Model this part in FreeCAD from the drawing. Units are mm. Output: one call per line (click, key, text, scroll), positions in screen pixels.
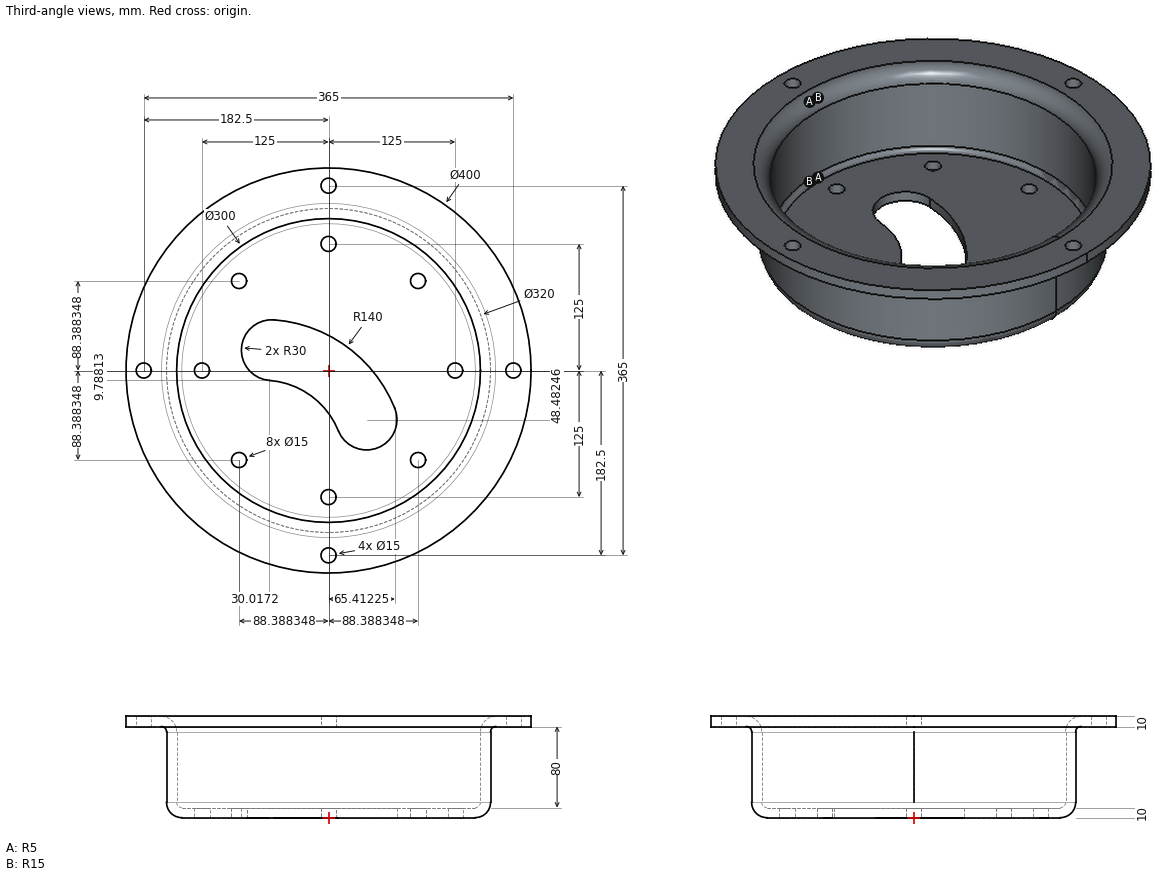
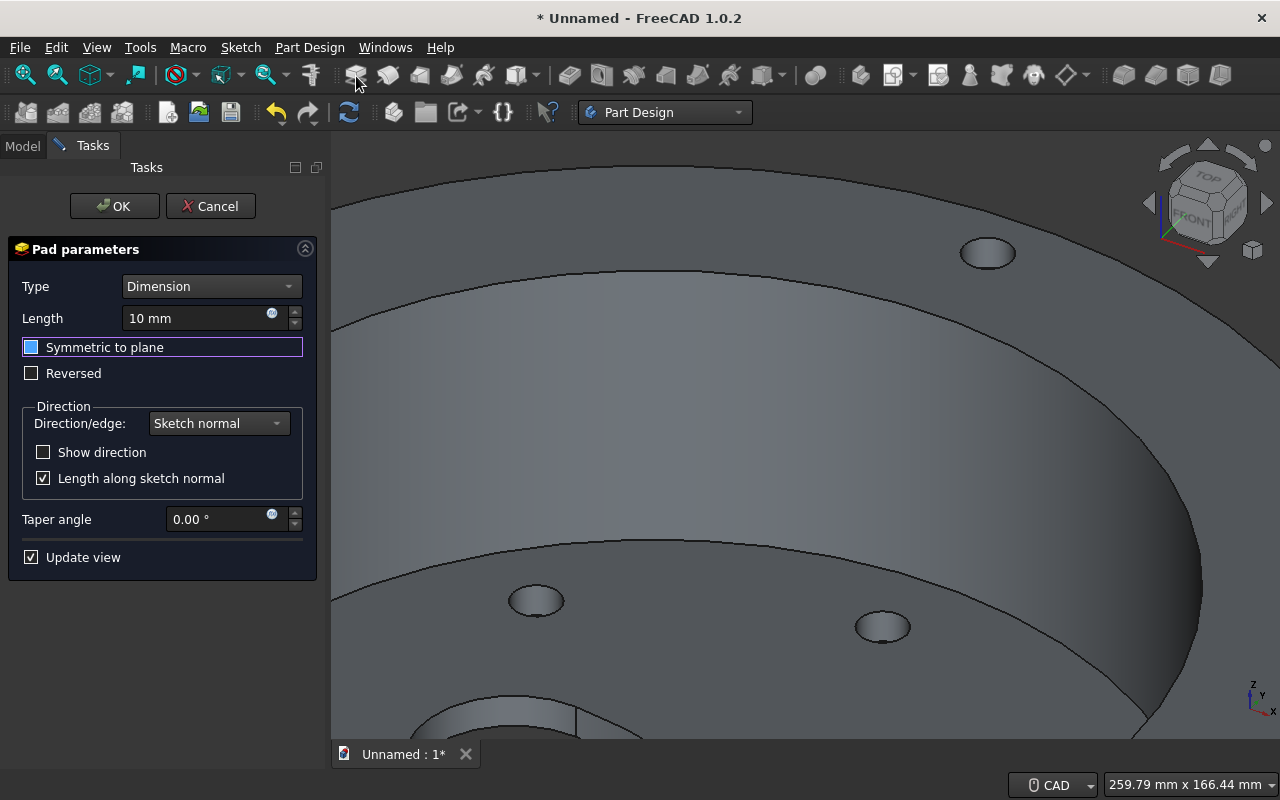
click(115, 206)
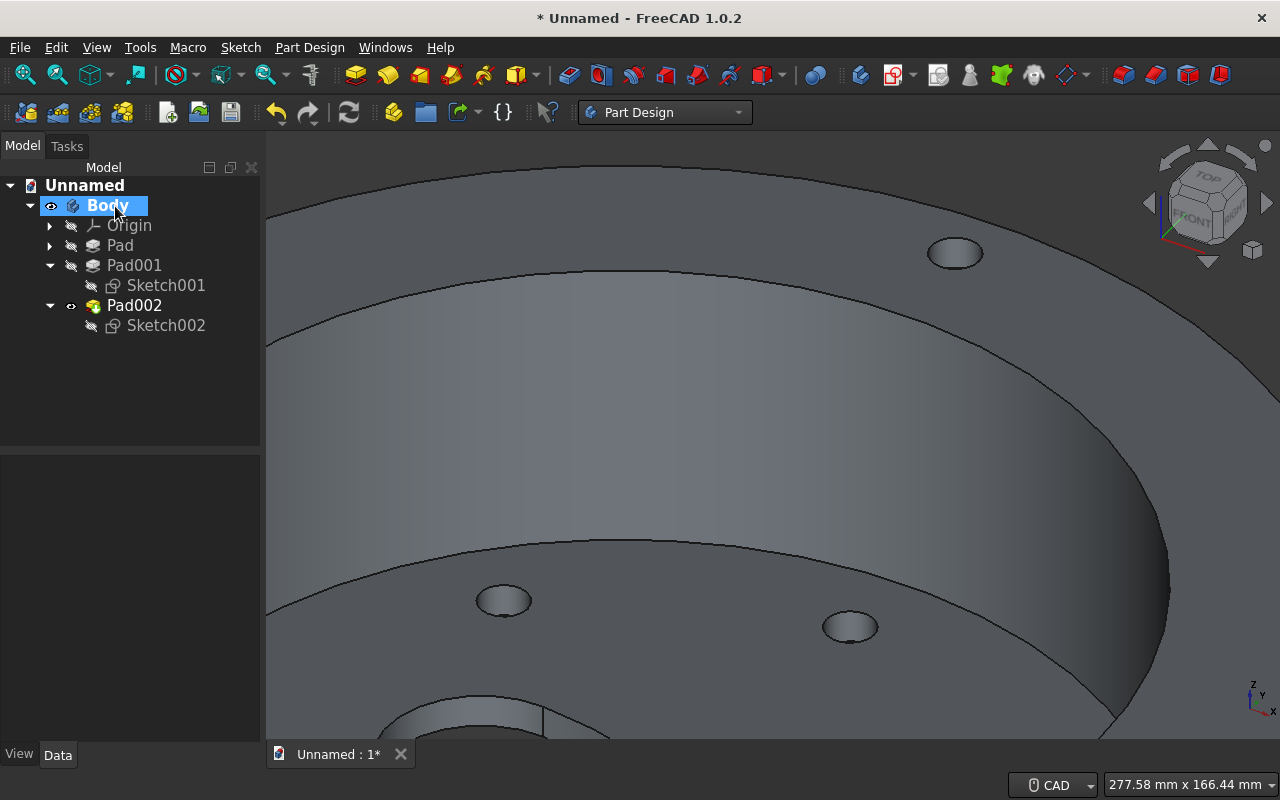
click(26, 76)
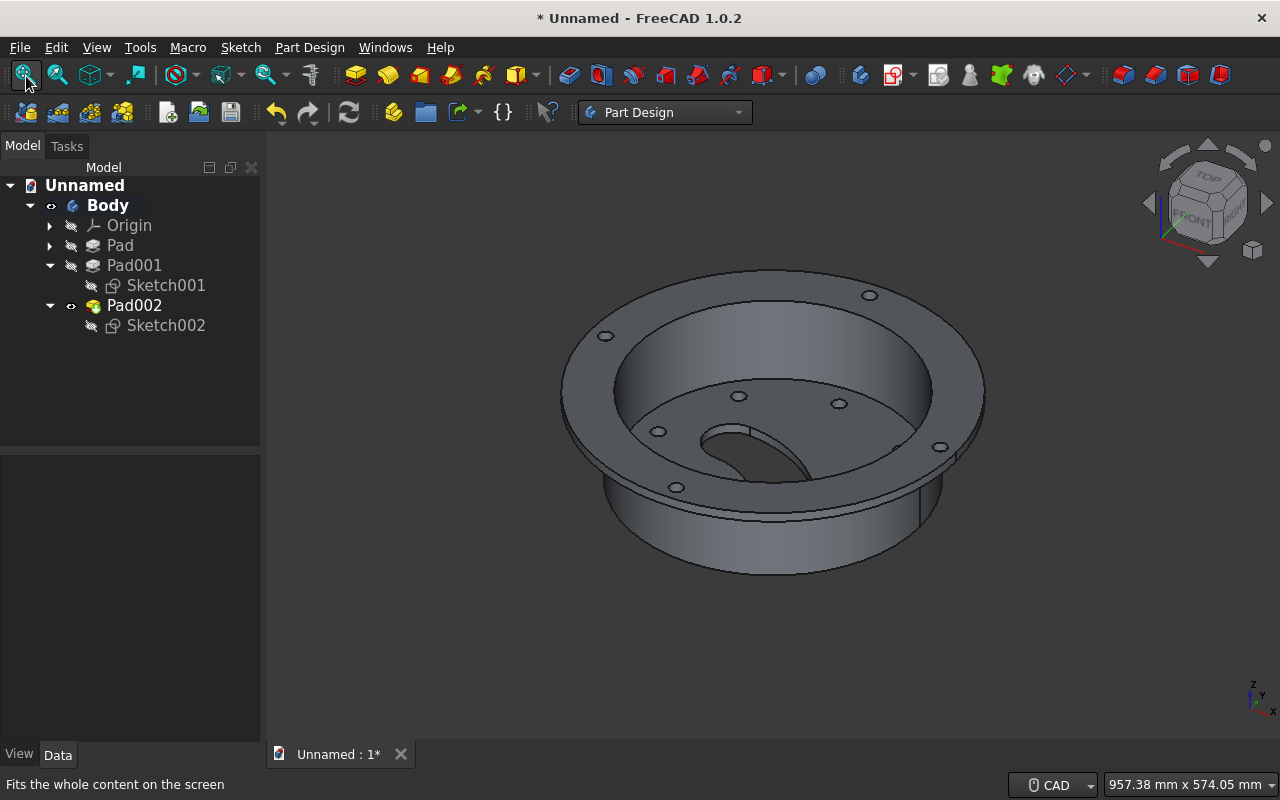
key(0)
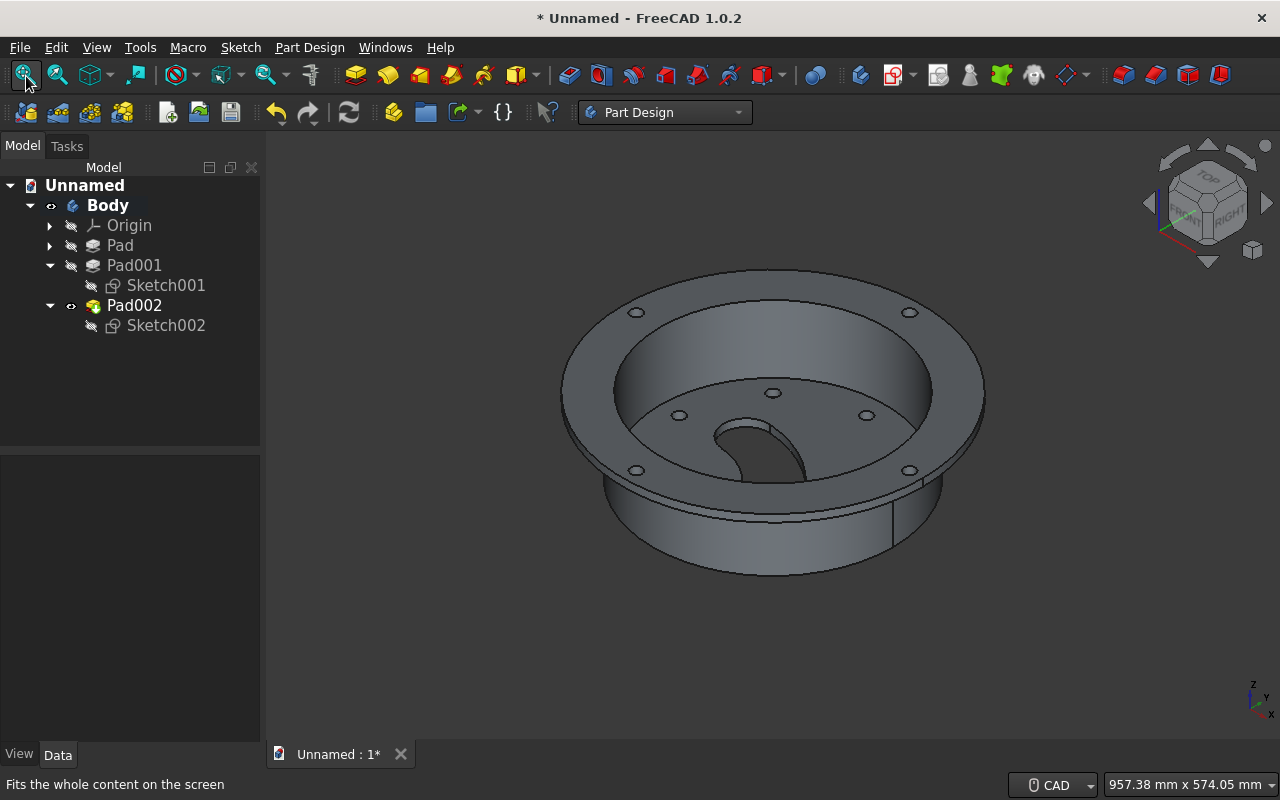
key(2)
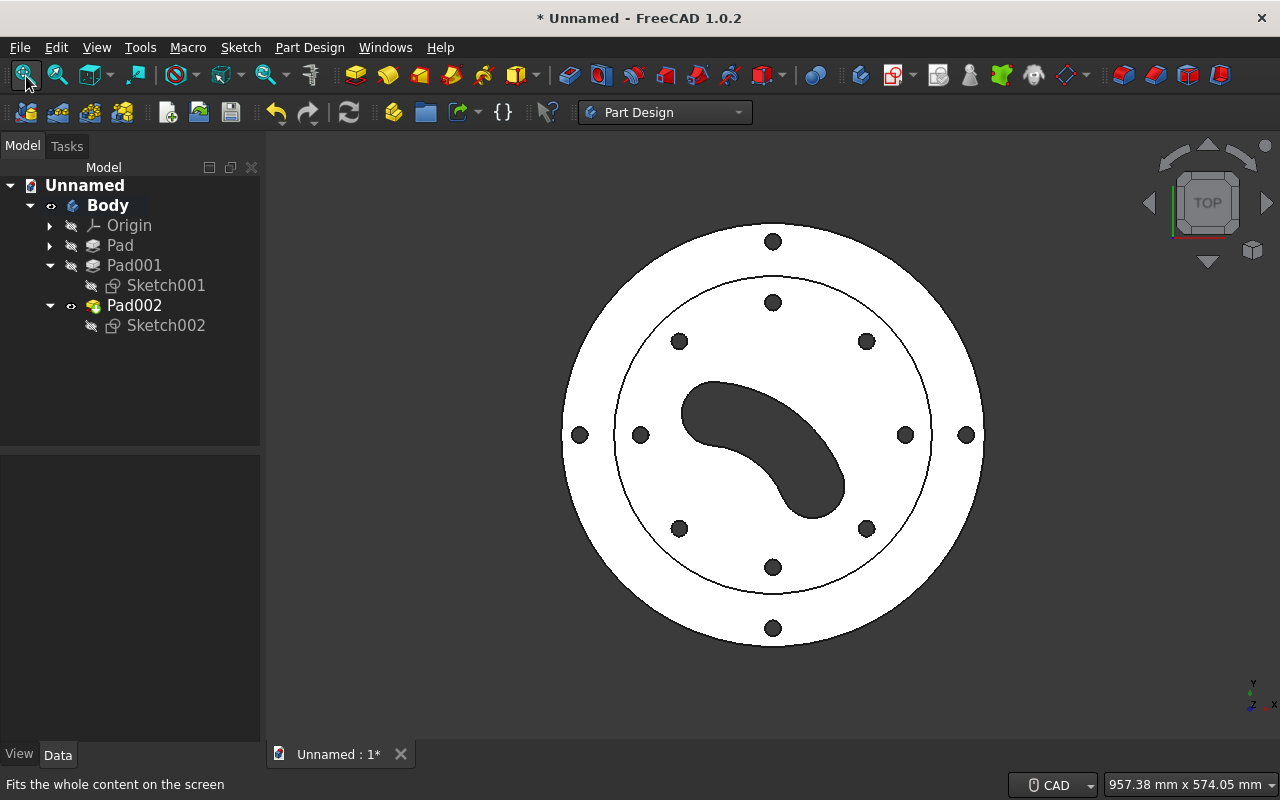
key(1)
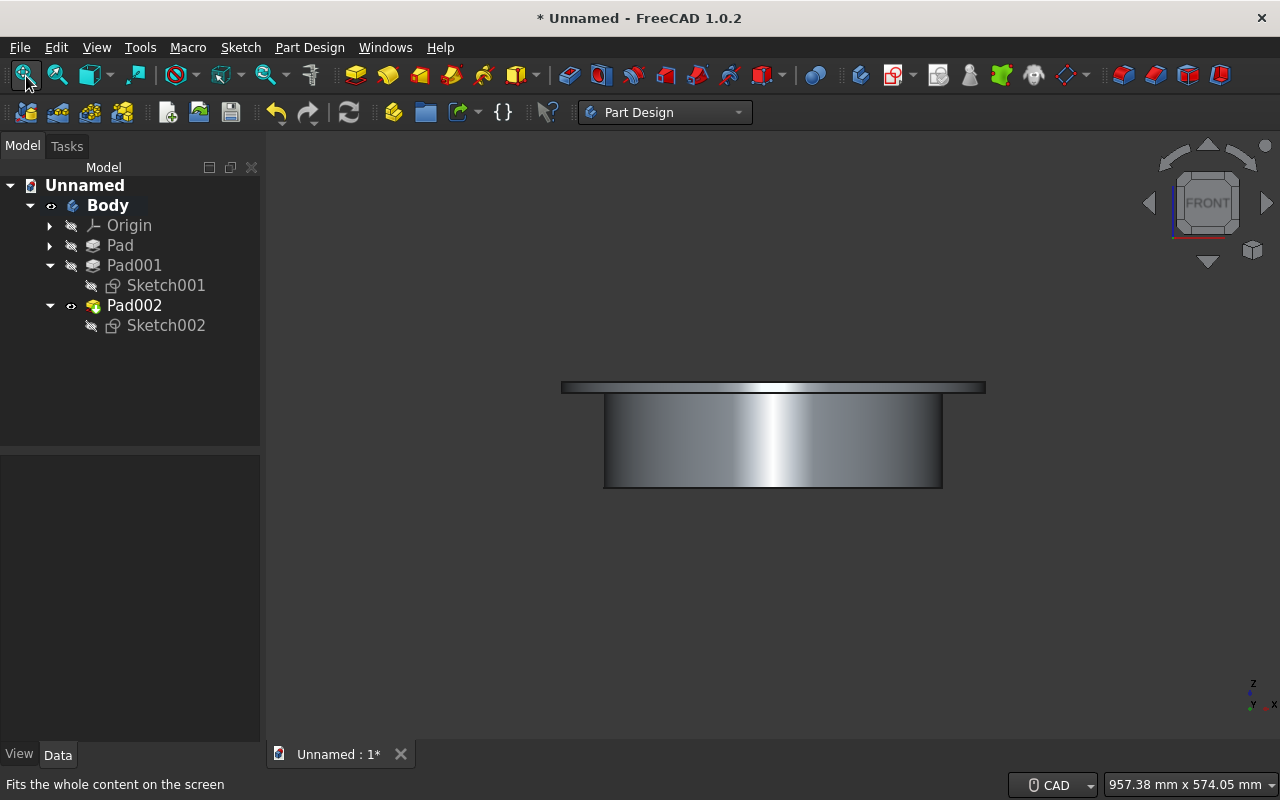
click(26, 76)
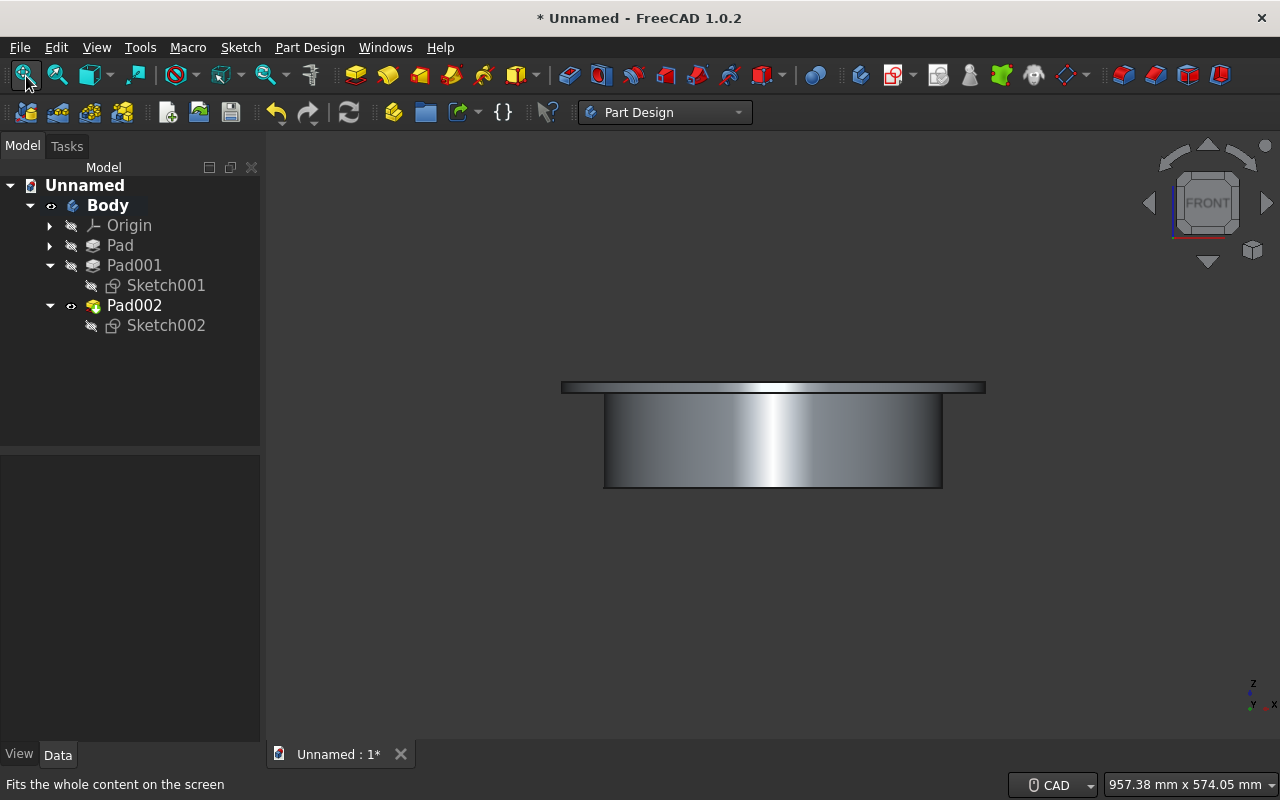
key(3)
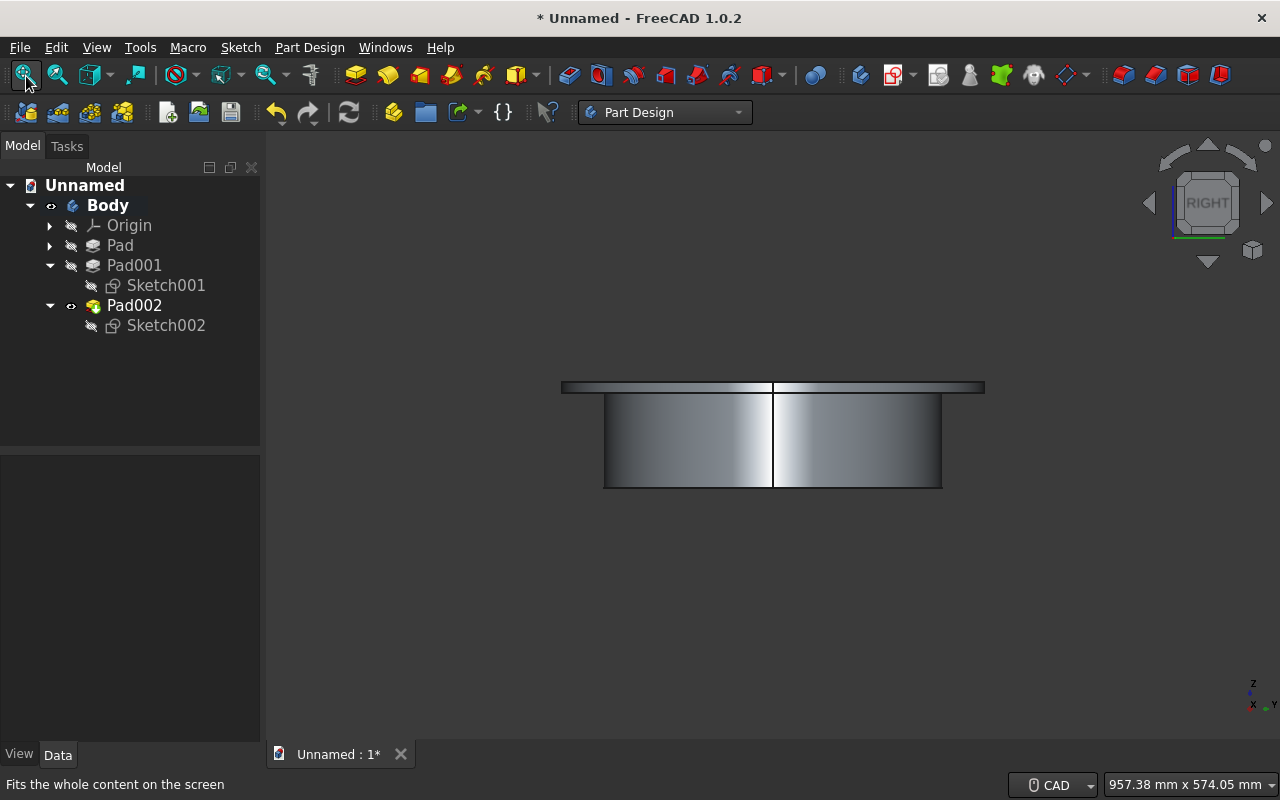
click(26, 76)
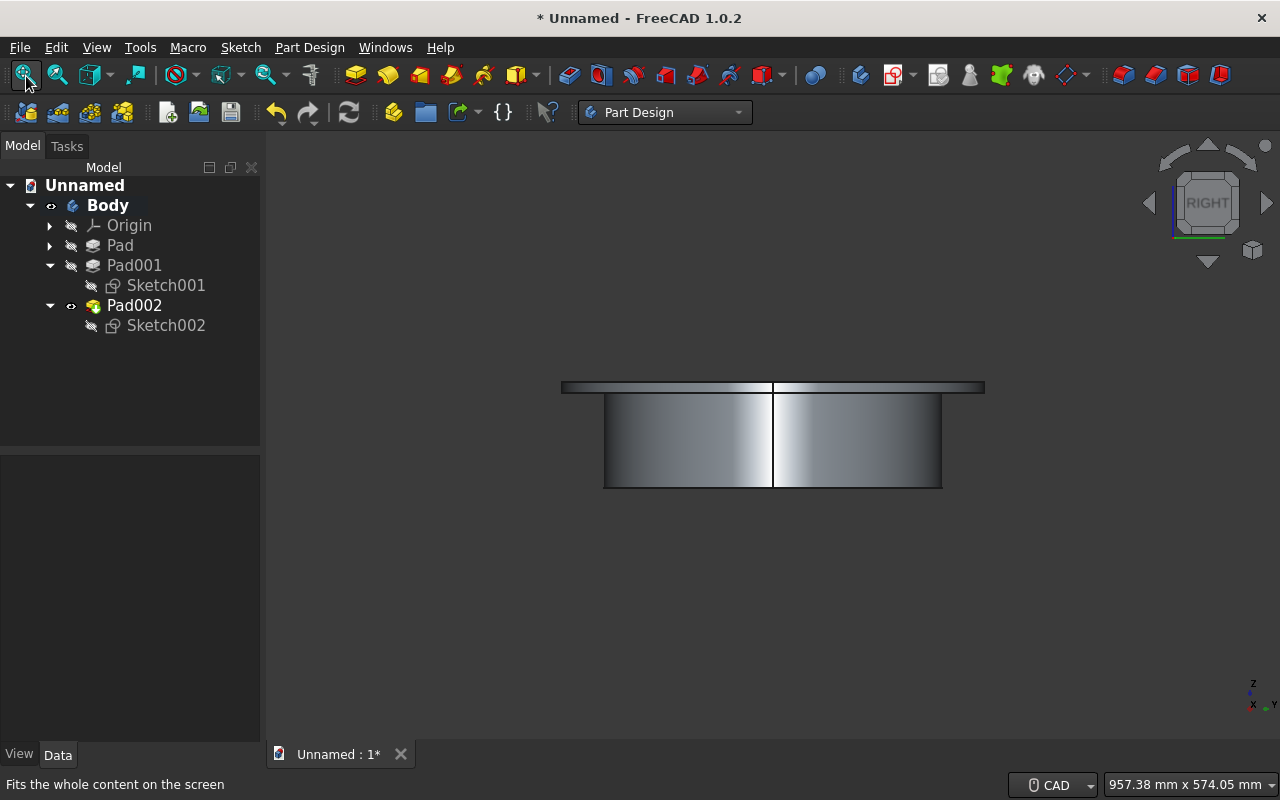
key(5)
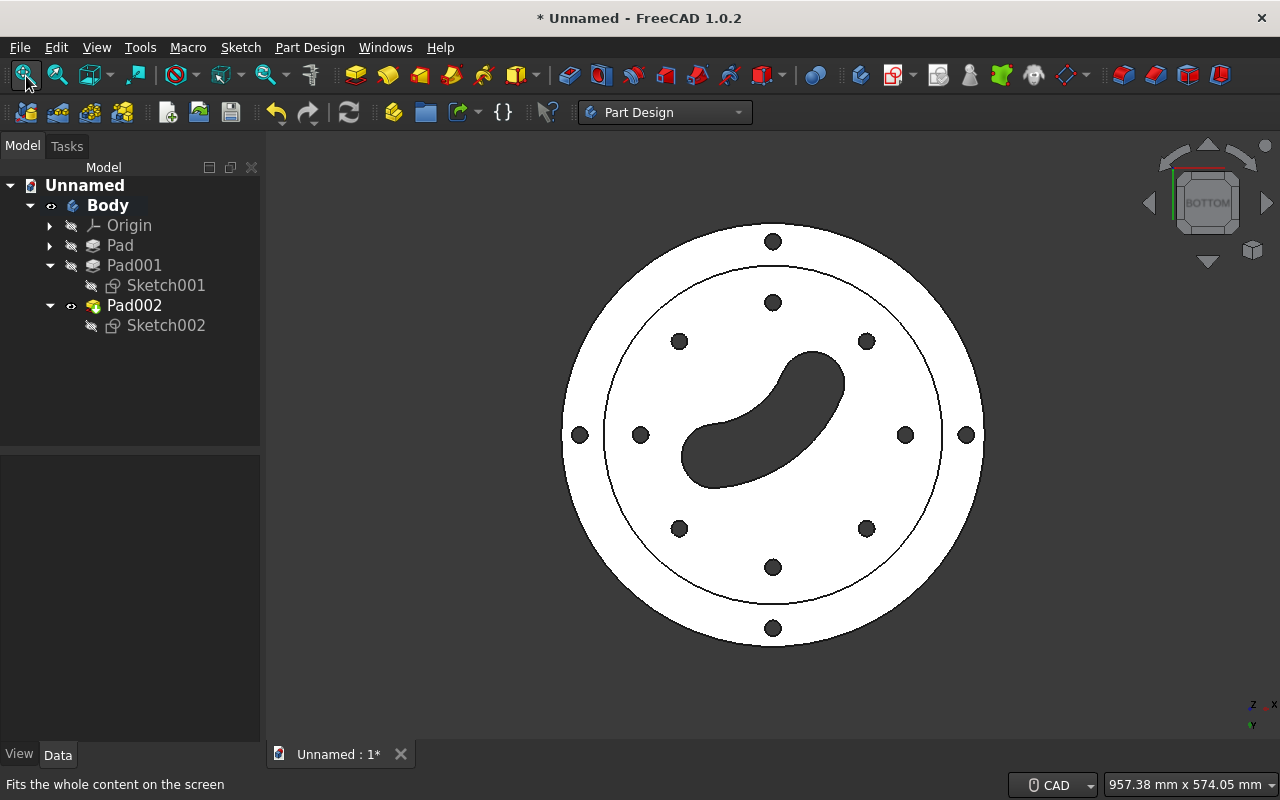
key(4)